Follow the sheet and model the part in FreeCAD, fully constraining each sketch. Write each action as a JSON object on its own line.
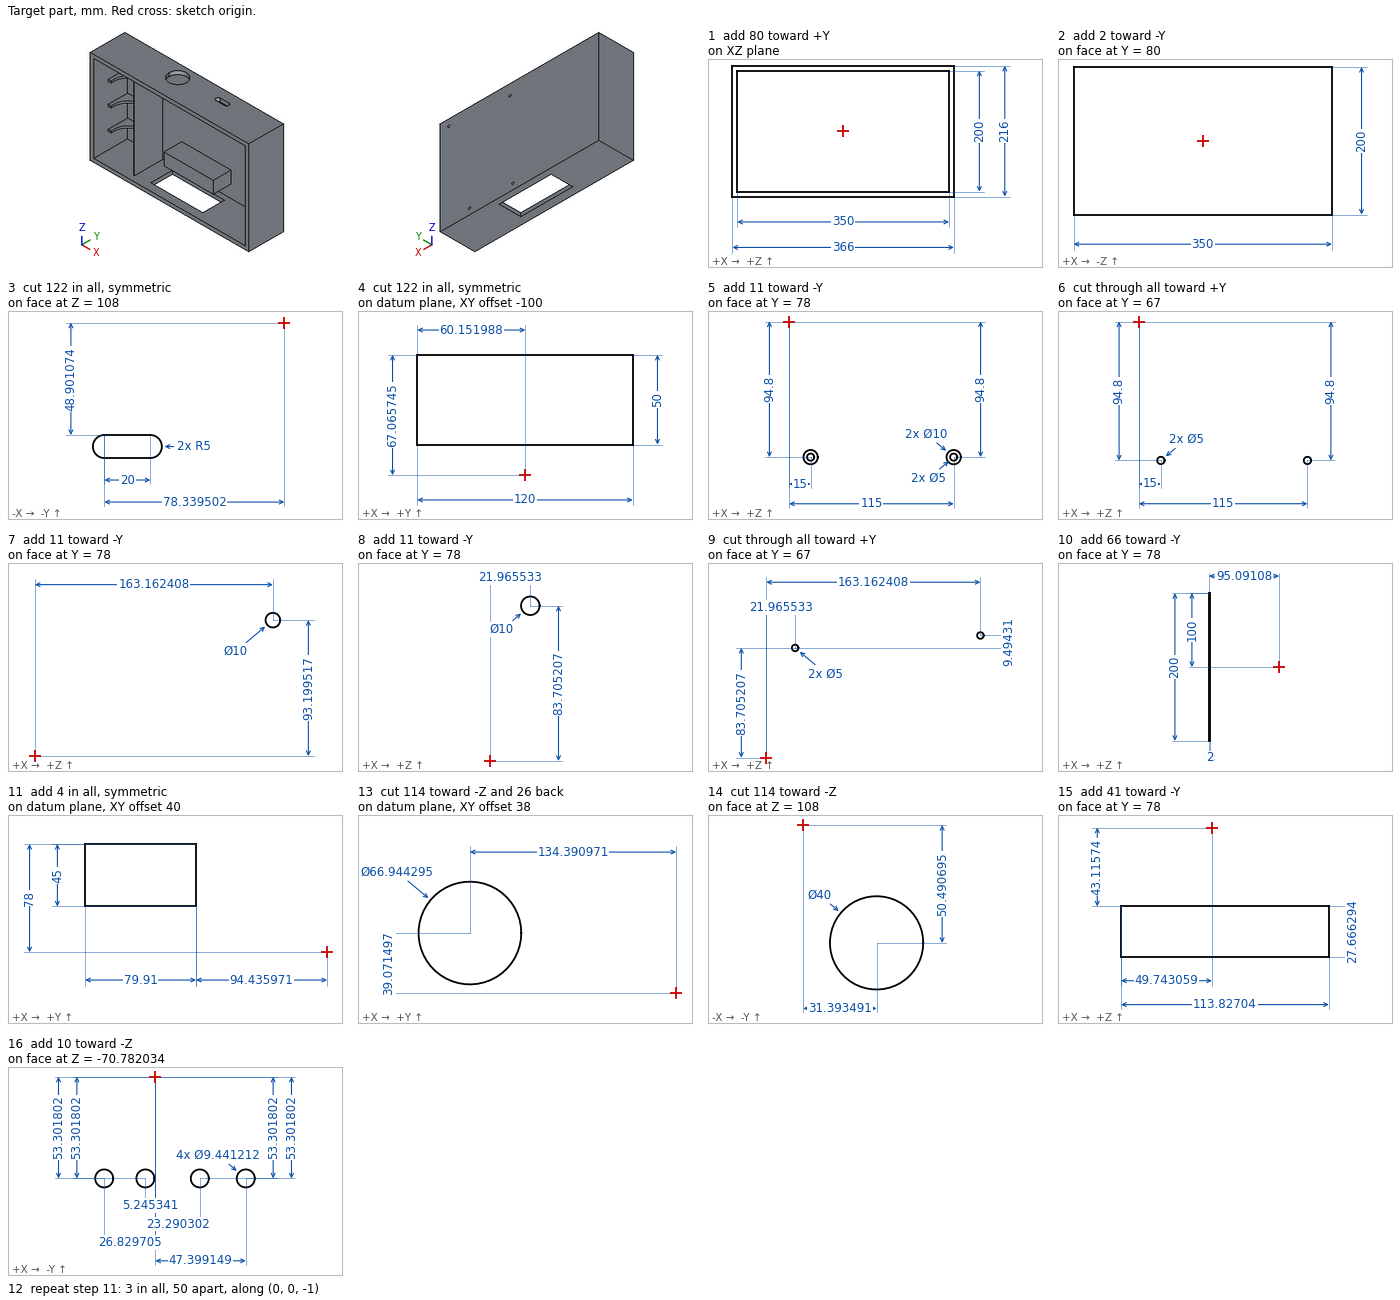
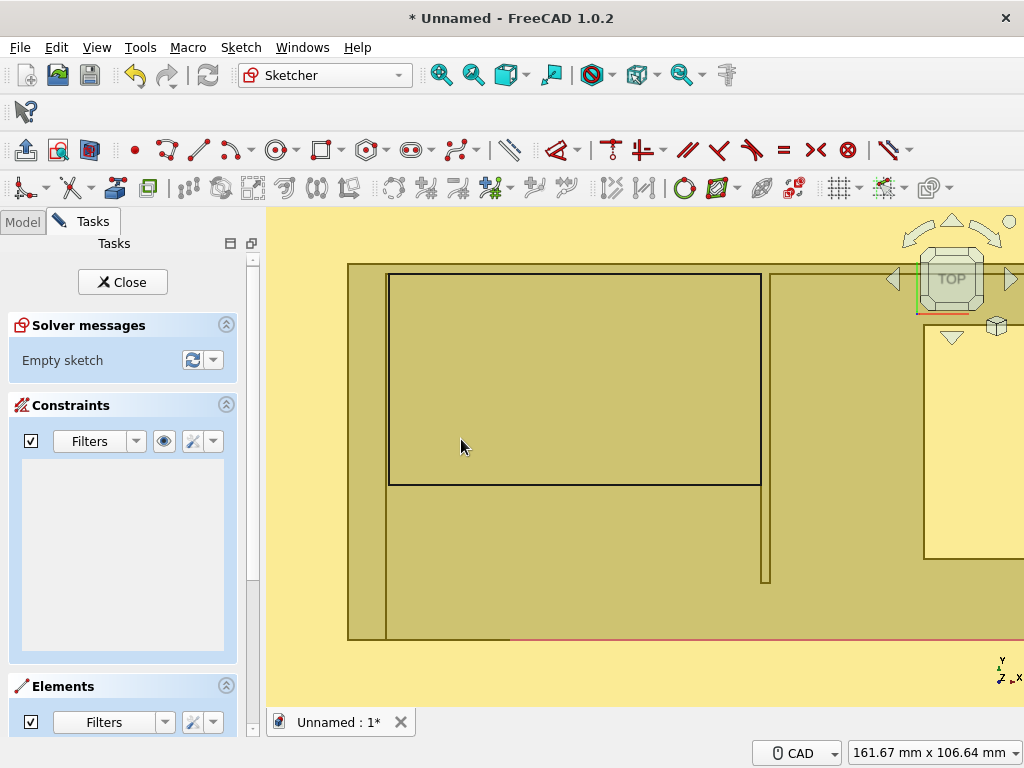
{"action": "key", "text": "g c"}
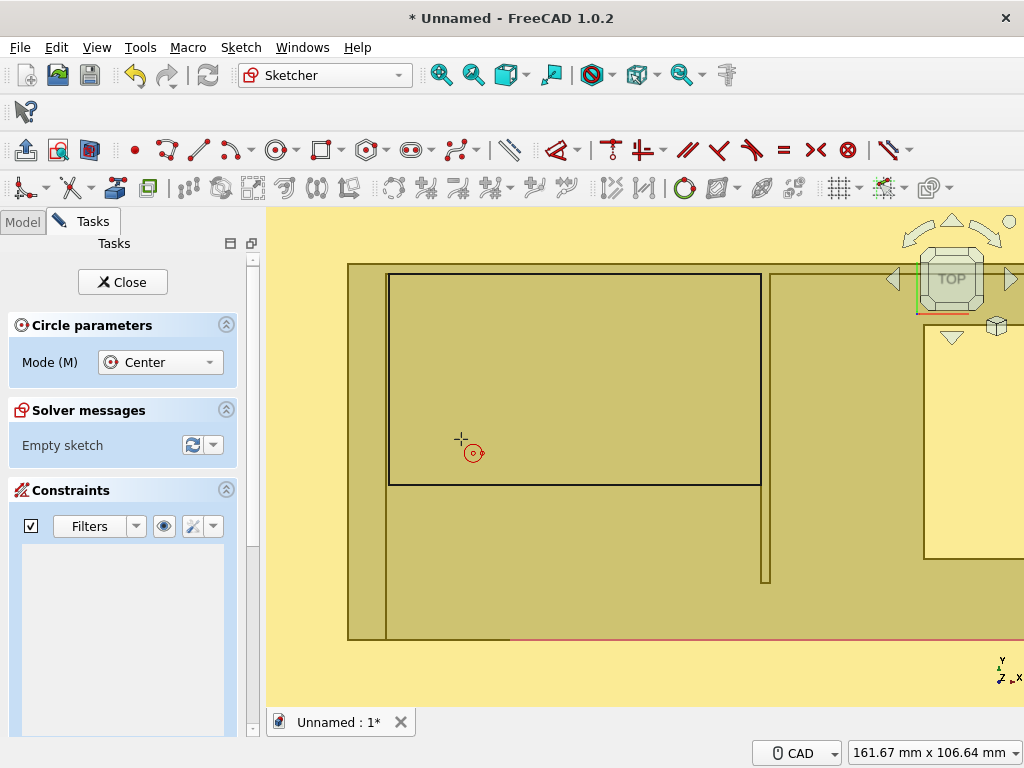
{"action": "left_click", "coordinate": [576, 456]}
{"action": "mouse_move", "coordinate": [687, 345]}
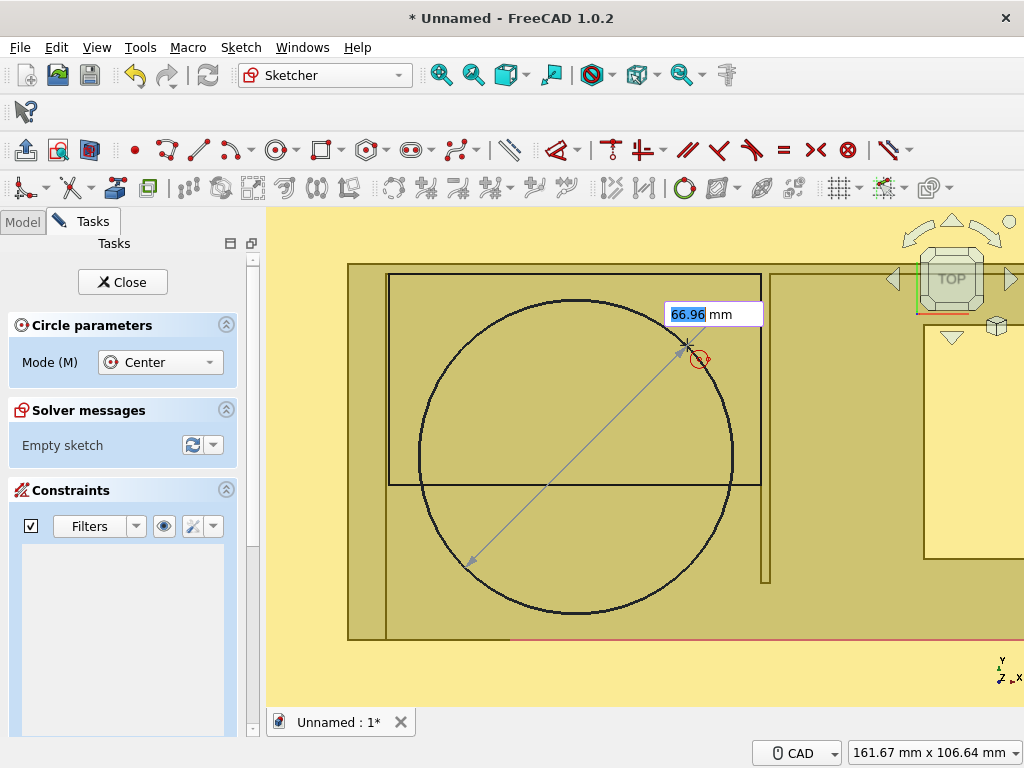
{"action": "type", "text": "66.944295"}
{"action": "key", "text": "Return"}
{"action": "key", "text": "Escape"}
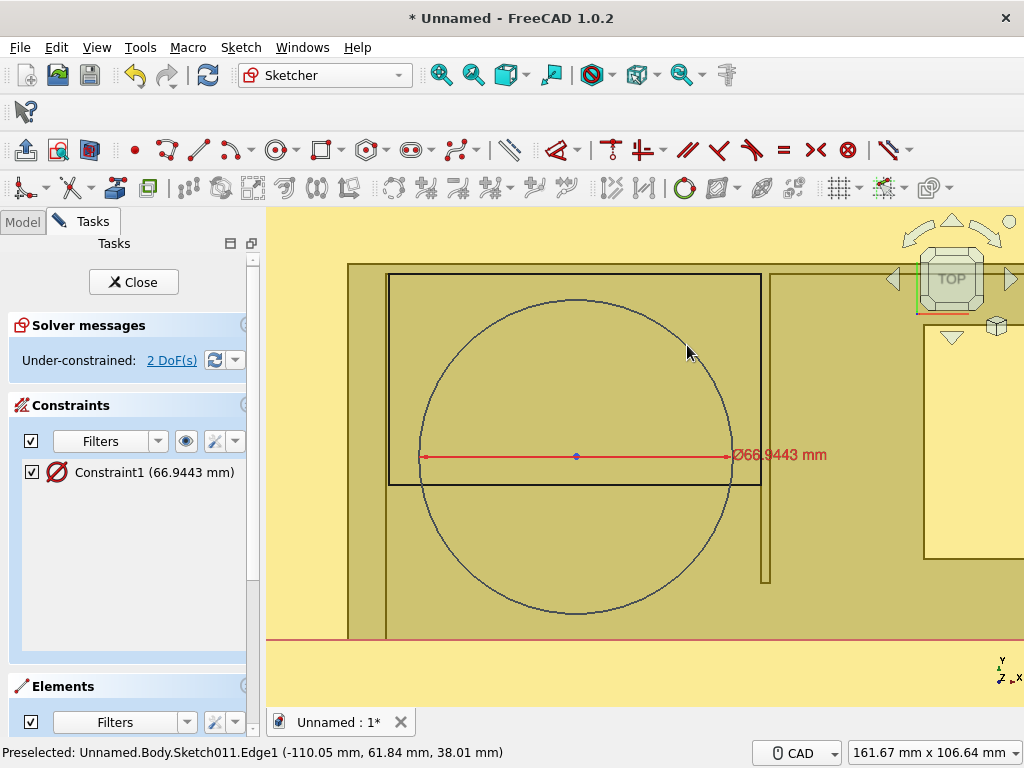
{"action": "key", "text": "d"}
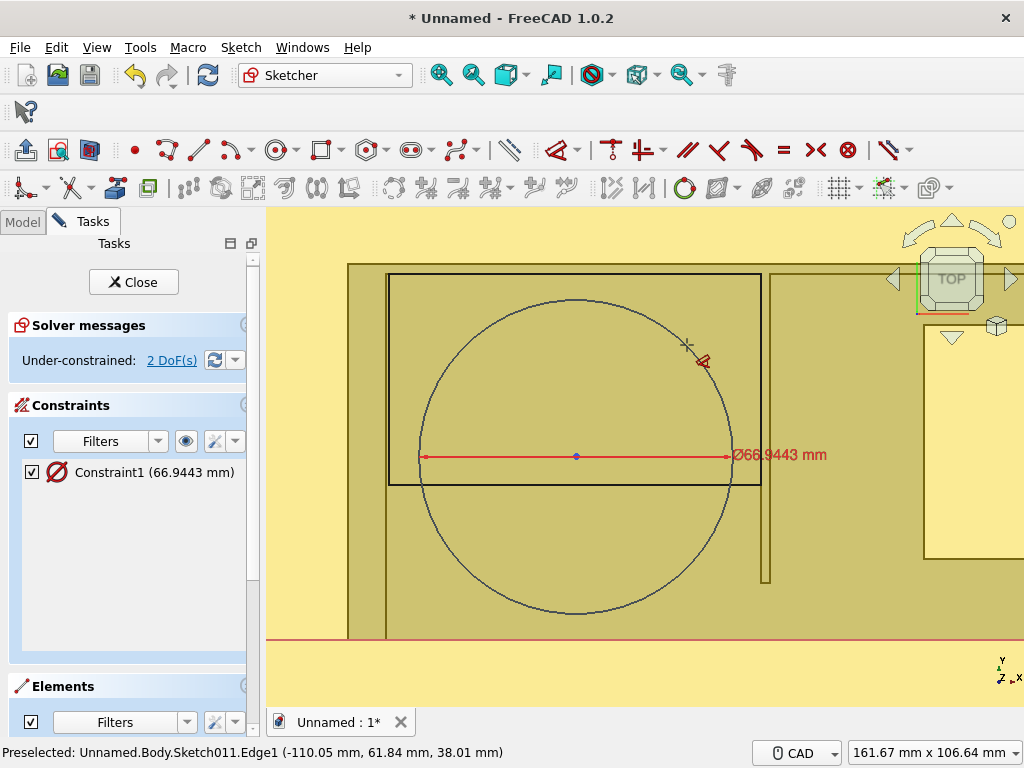
{"action": "left_click", "coordinate": [576, 457]}
{"action": "left_click", "coordinate": [542, 548]}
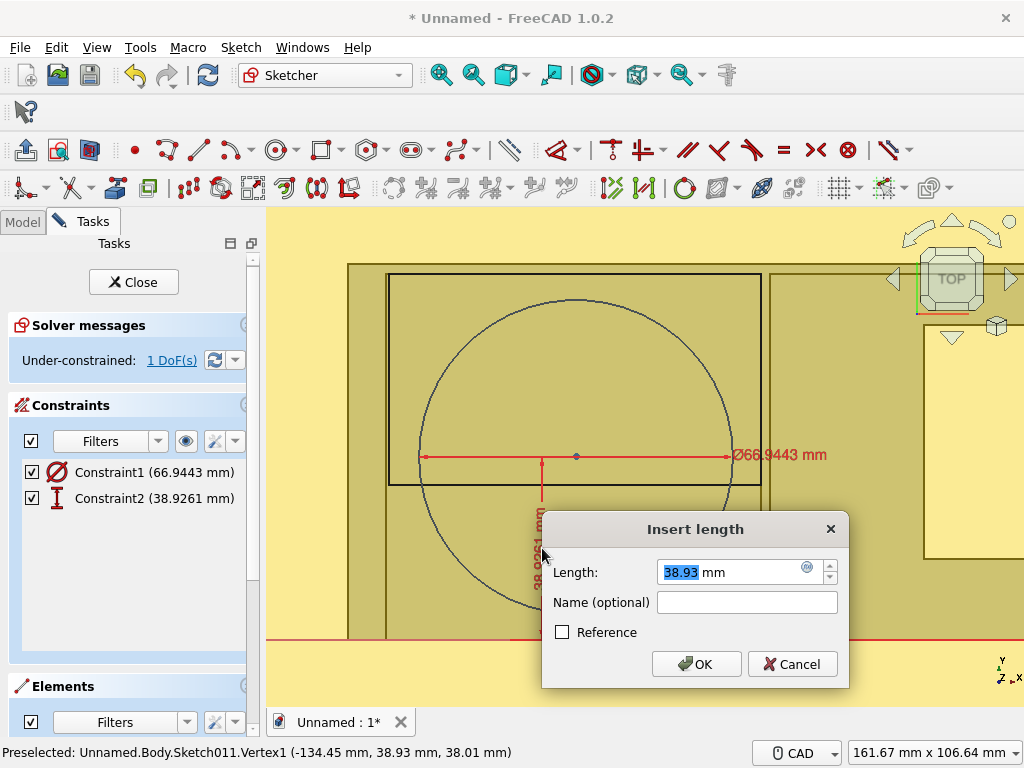
{"action": "type", "text": "39.071497"}
{"action": "key", "text": "Return"}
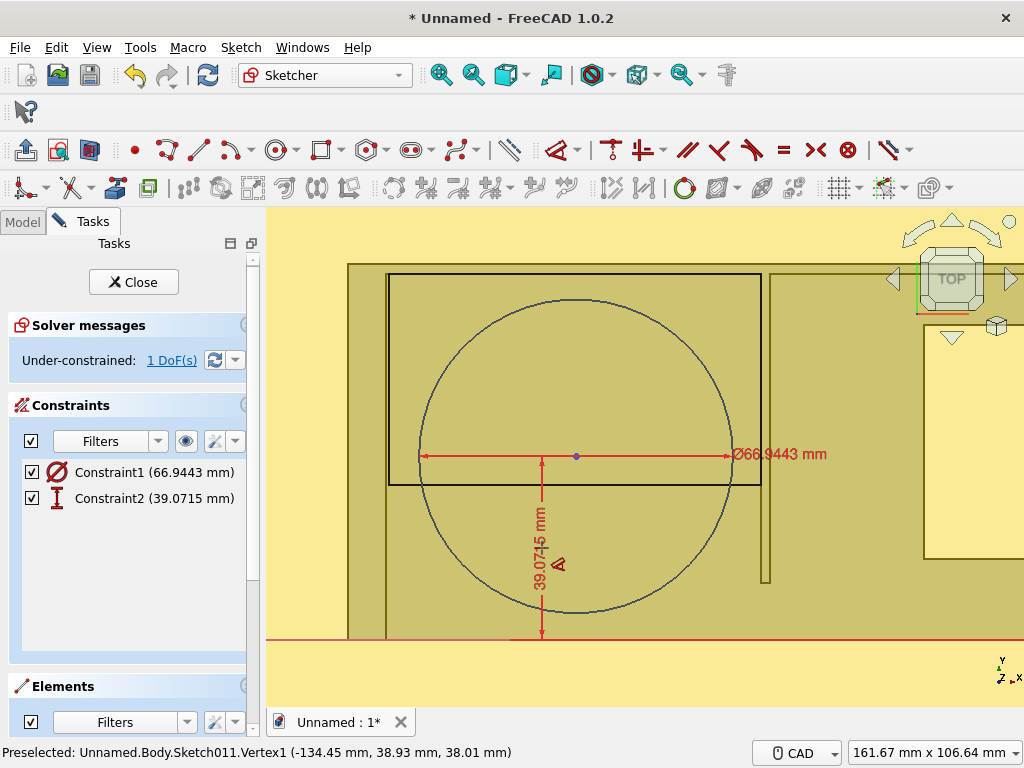
{"action": "left_click", "coordinate": [576, 456]}
{"action": "left_click", "coordinate": [718, 674]}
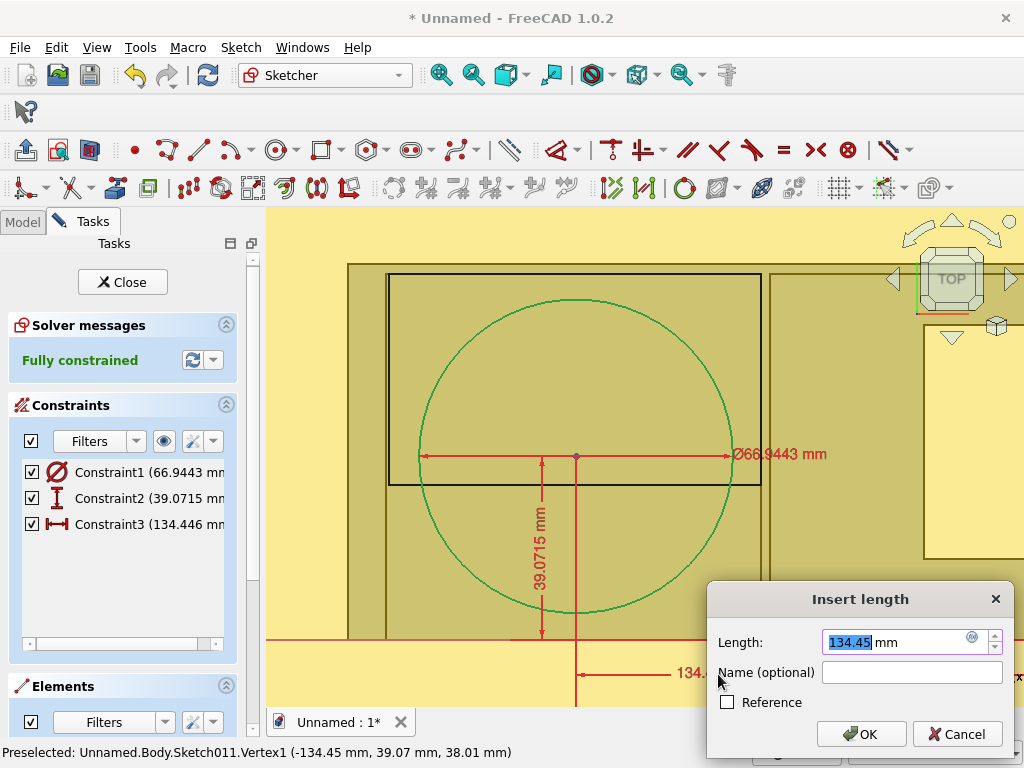
{"action": "type", "text": "134.390971"}
{"action": "key", "text": "Return"}
{"action": "key", "text": "Escape"}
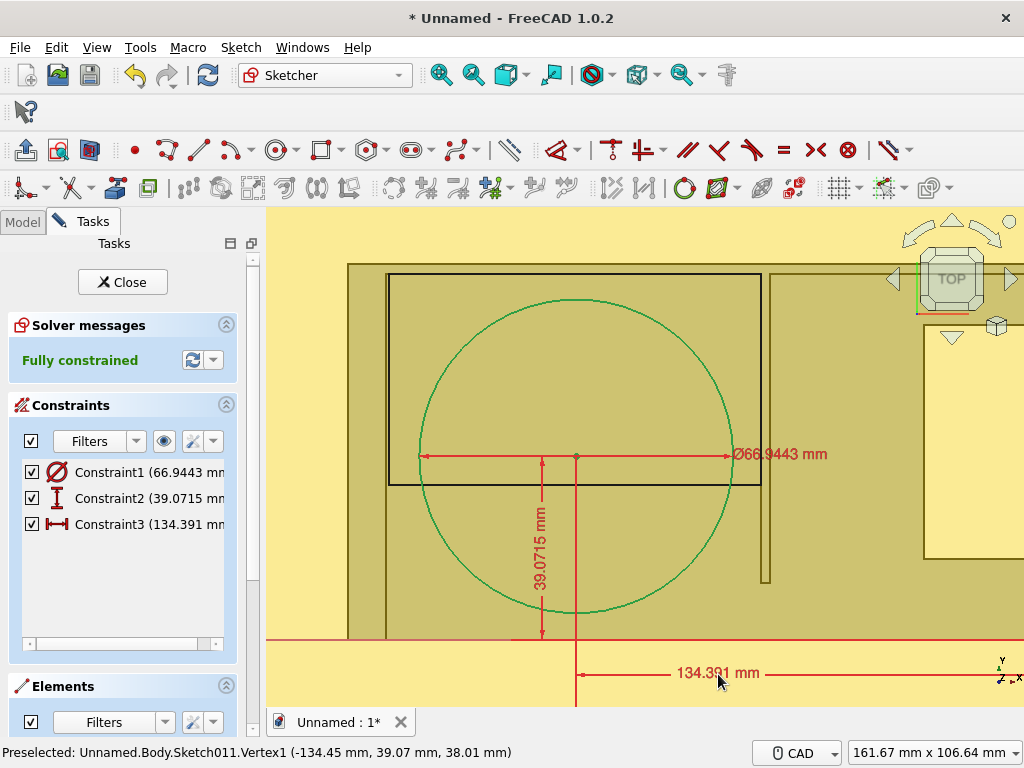
{"action": "left_click", "coordinate": [123, 282]}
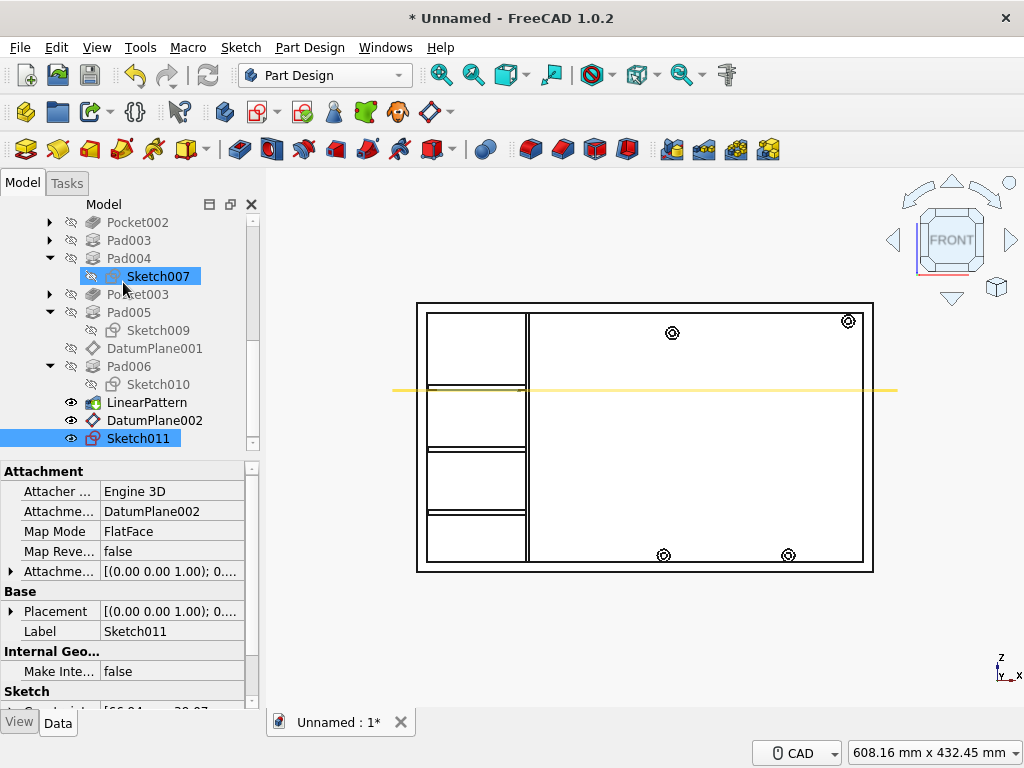
{"action": "left_click", "coordinate": [240, 150]}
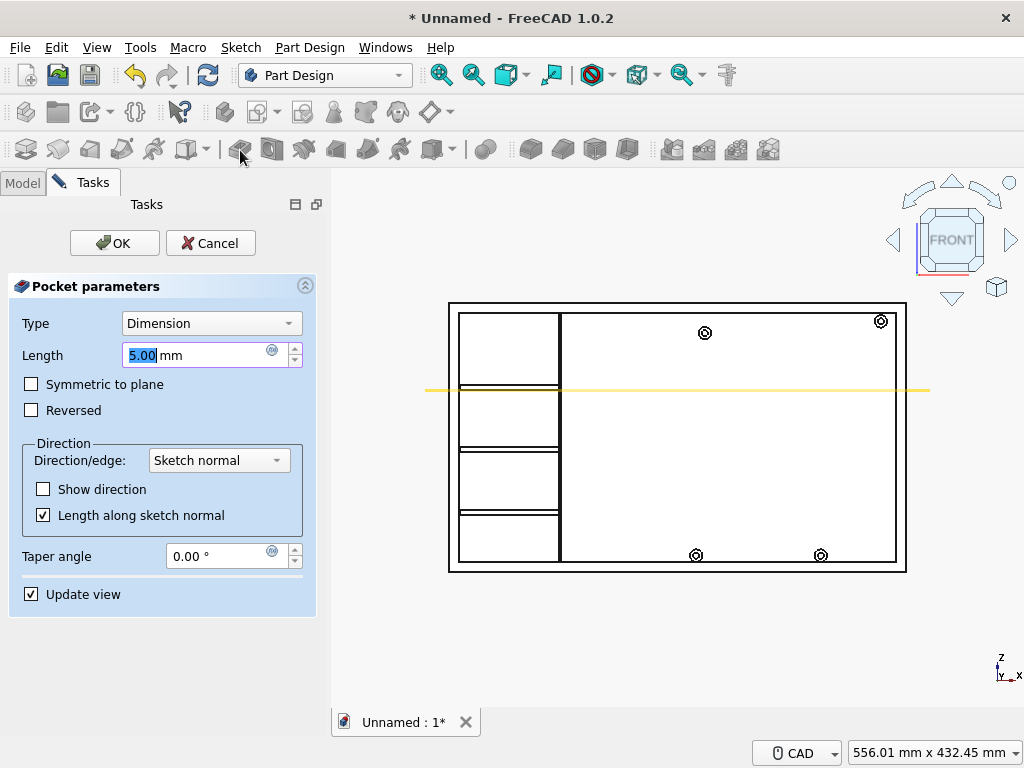
{"action": "left_click", "coordinate": [212, 324]}